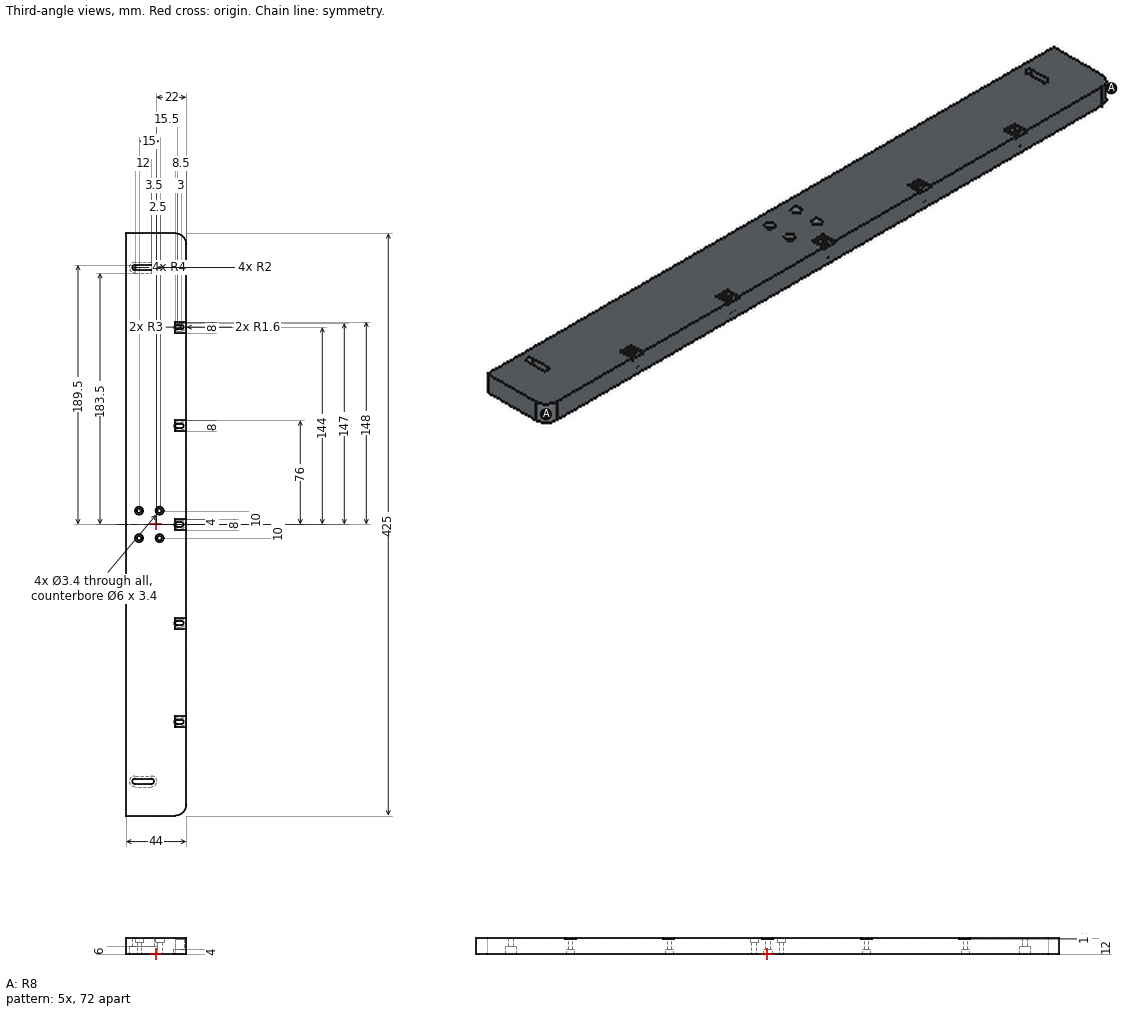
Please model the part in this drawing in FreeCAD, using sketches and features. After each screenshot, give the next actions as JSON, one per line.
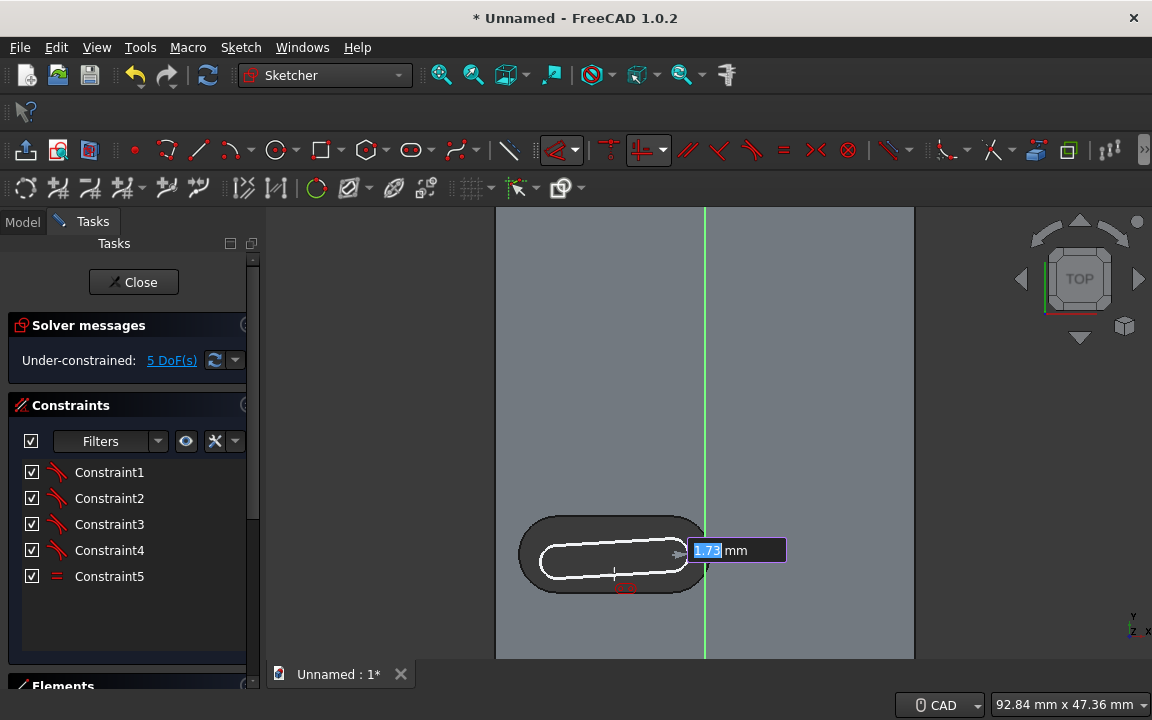
{"action": "left_click", "coordinate": [614, 574]}
{"action": "key", "text": "Escape"}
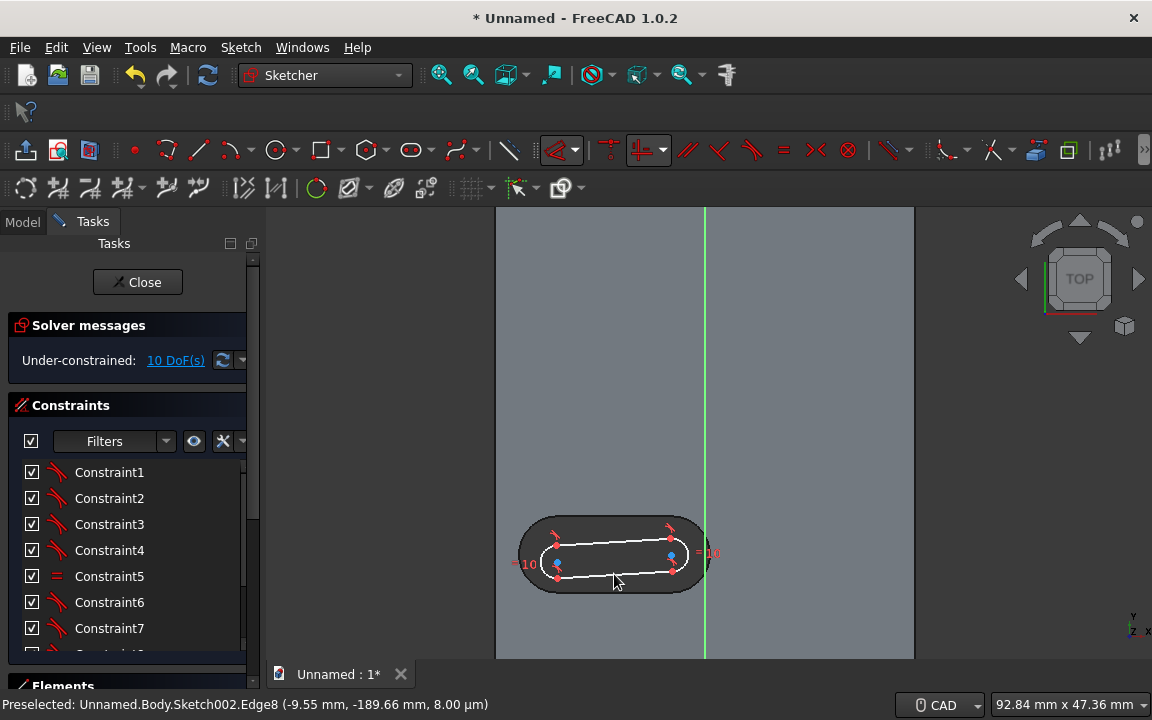
{"action": "scroll", "coordinate": [642, 567], "scroll_direction": "down", "scroll_amount": 13}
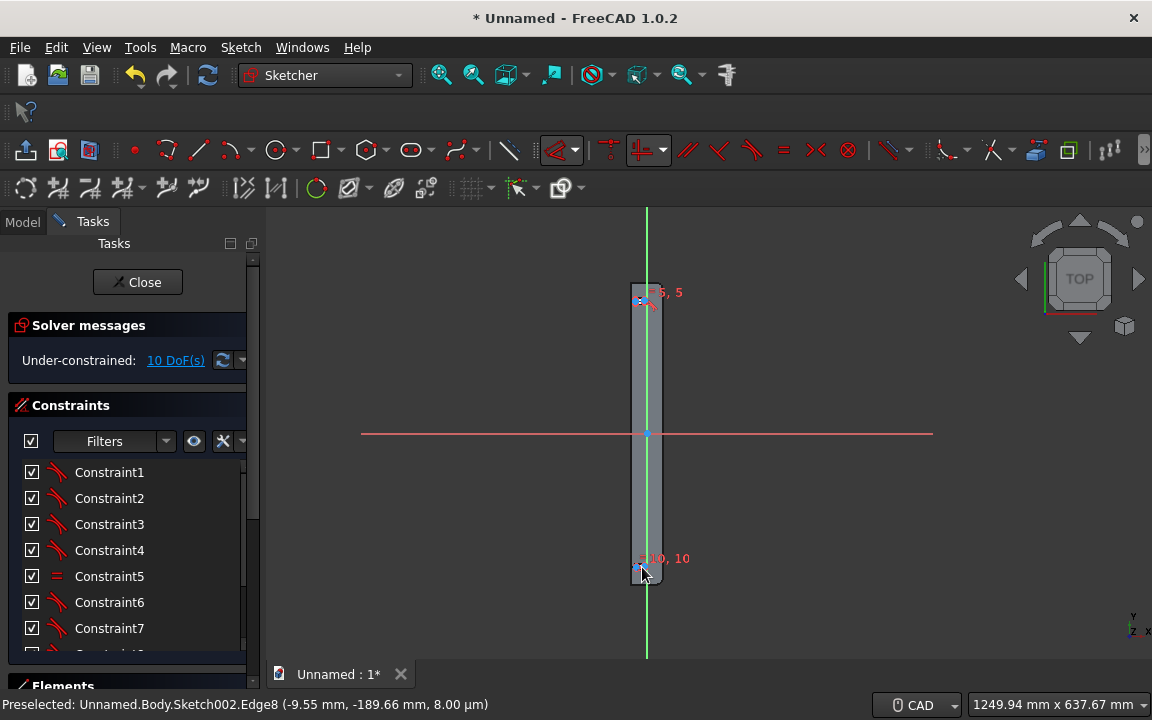
{"action": "scroll", "coordinate": [638, 300], "scroll_direction": "up", "scroll_amount": 9}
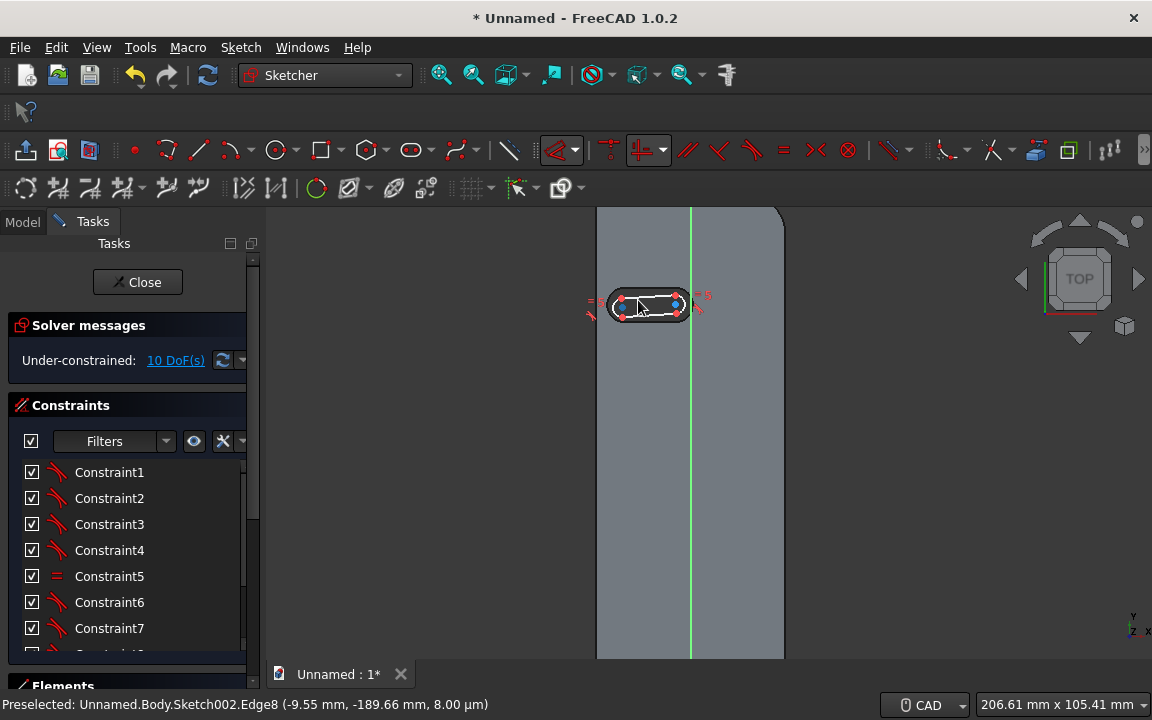
{"action": "left_click", "coordinate": [638, 298]}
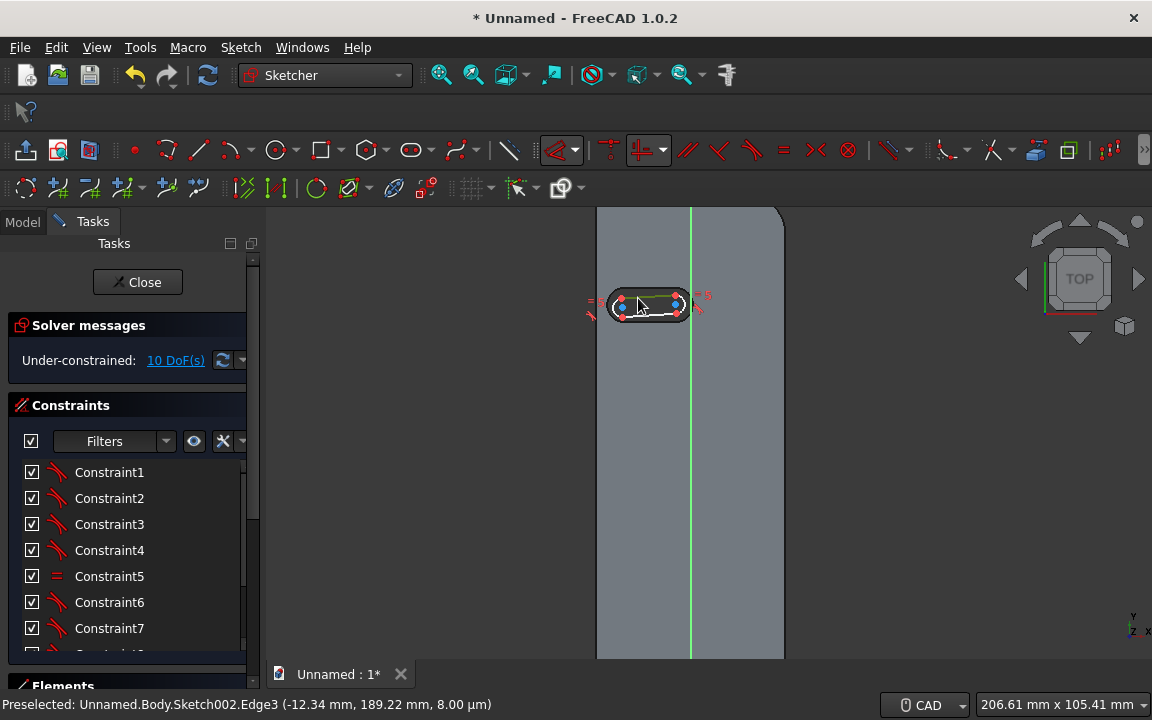
{"action": "left_click", "coordinate": [666, 150]}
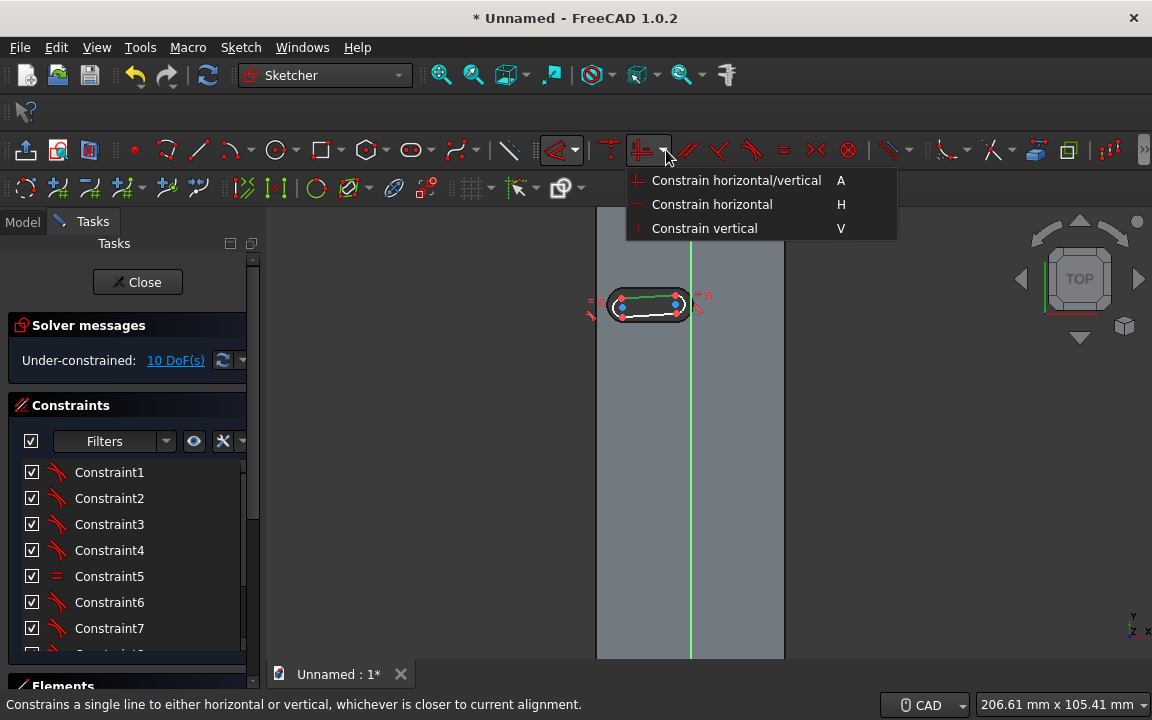
{"action": "left_click", "coordinate": [762, 204]}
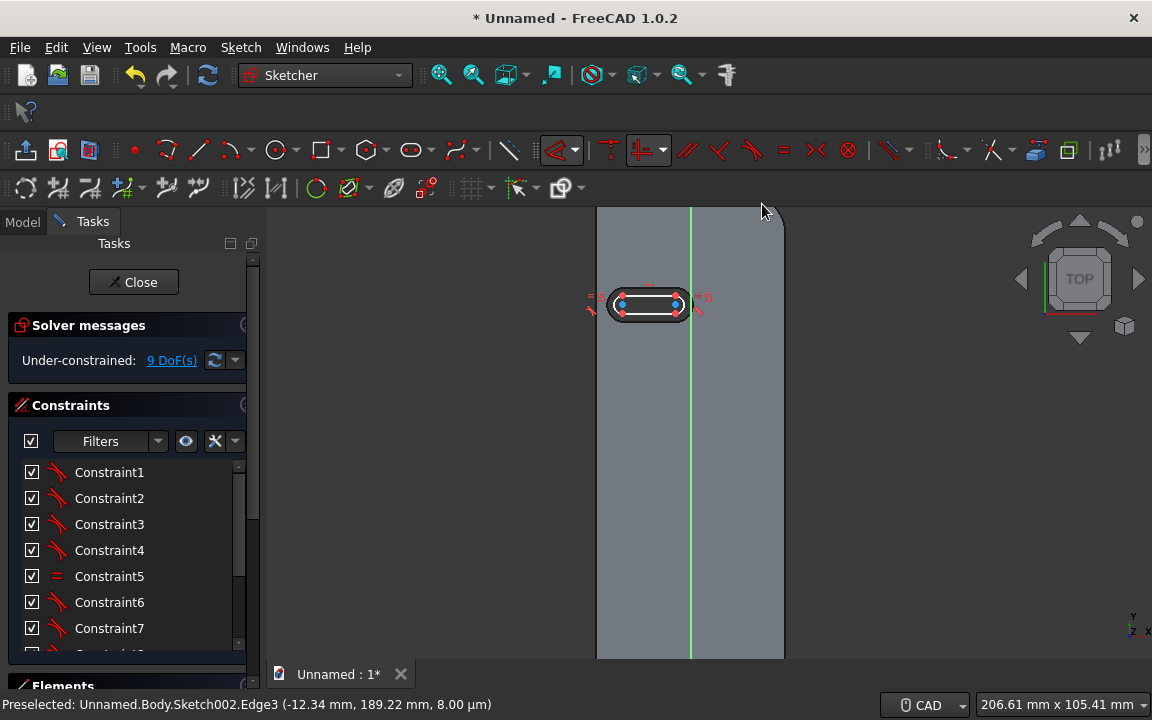
{"action": "scroll", "coordinate": [638, 299], "scroll_direction": "down", "scroll_amount": 9}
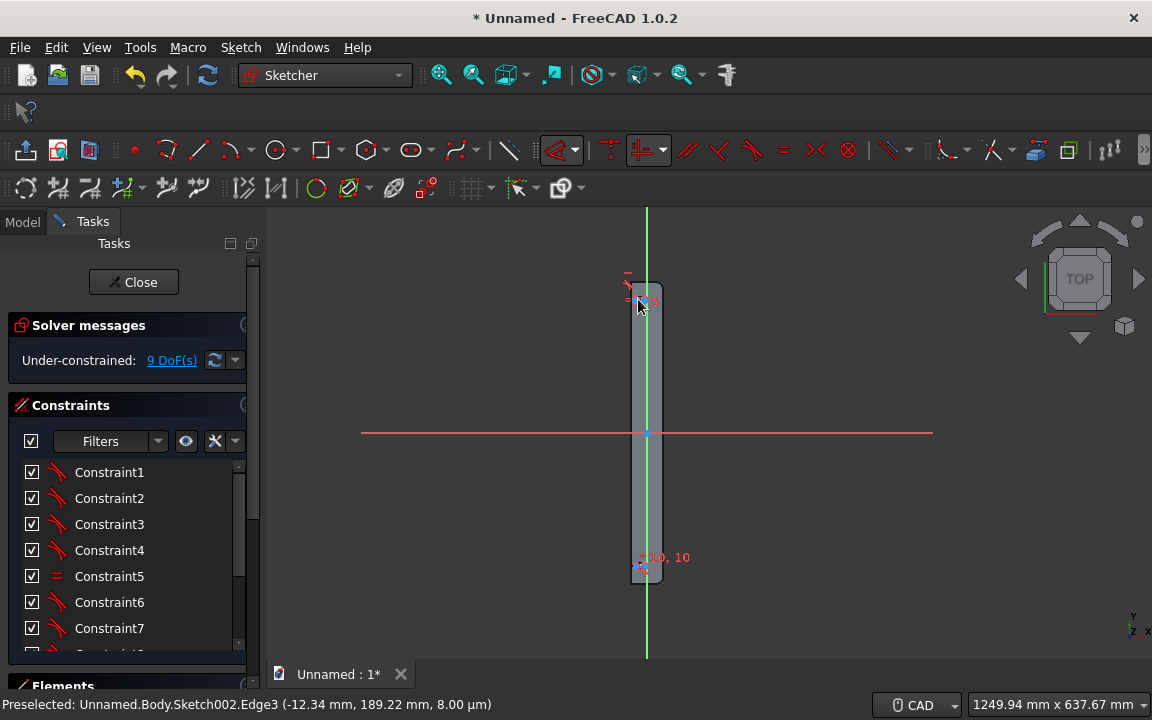
{"action": "scroll", "coordinate": [639, 565], "scroll_direction": "up", "scroll_amount": 9}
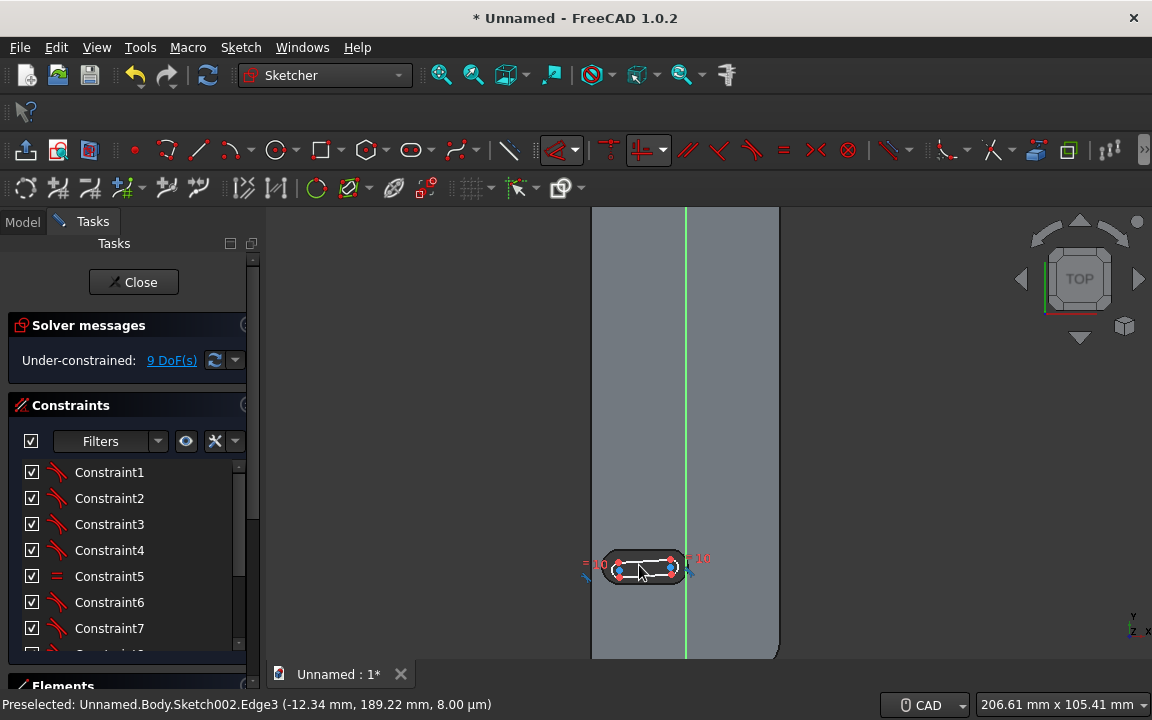
{"action": "left_click", "coordinate": [634, 562]}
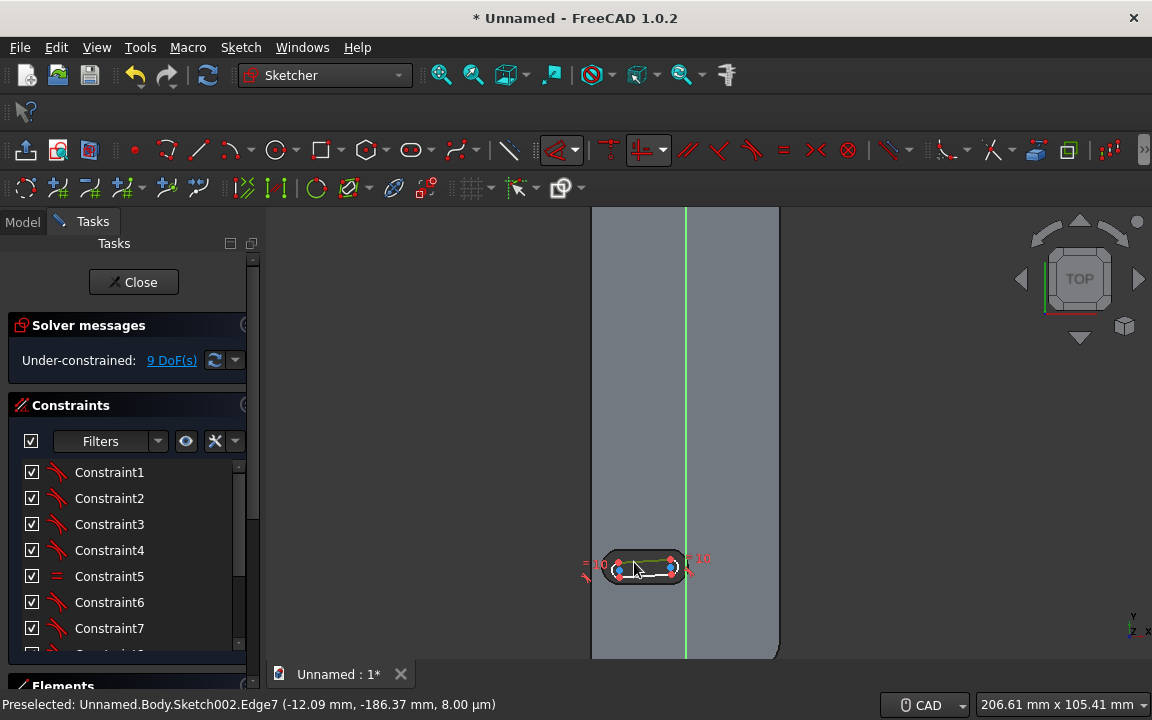
{"action": "key", "text": "h"}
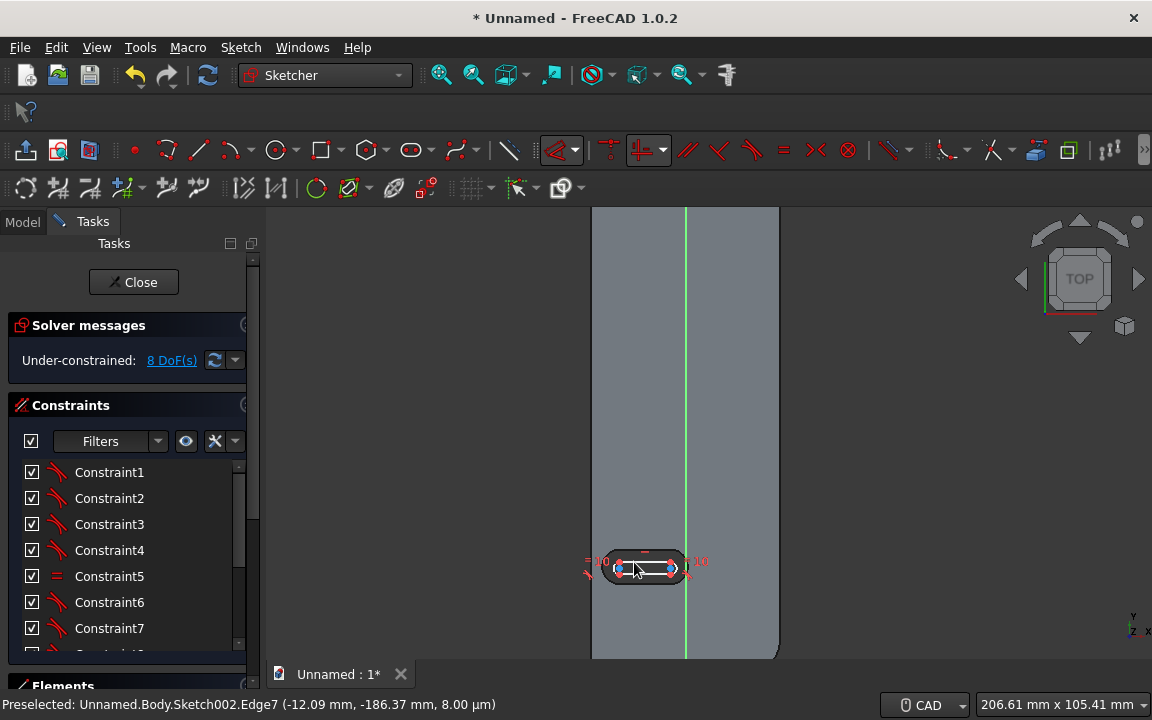
{"action": "scroll", "coordinate": [639, 566], "scroll_direction": "down", "scroll_amount": 9}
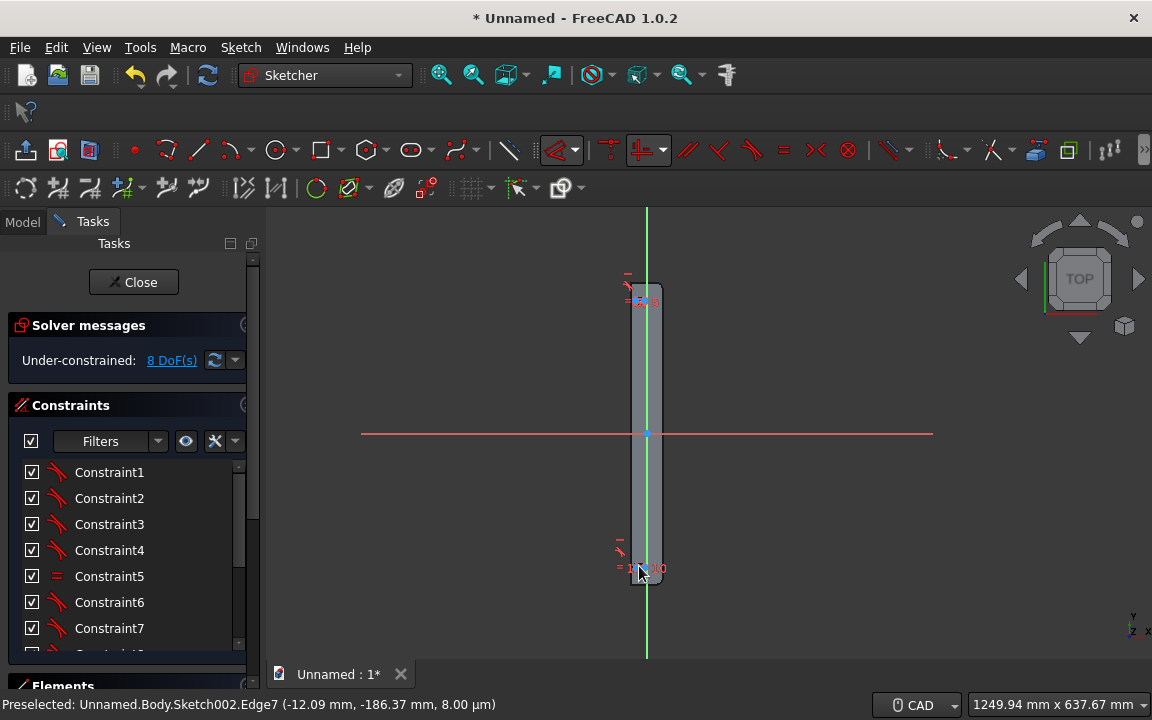
{"action": "scroll", "coordinate": [634, 301], "scroll_direction": "up", "scroll_amount": 12}